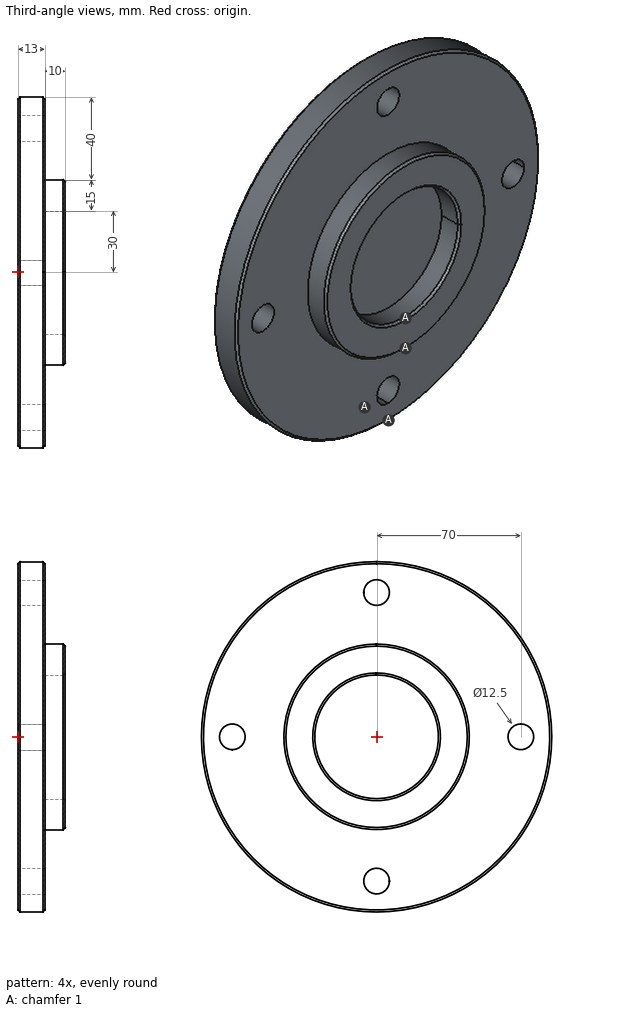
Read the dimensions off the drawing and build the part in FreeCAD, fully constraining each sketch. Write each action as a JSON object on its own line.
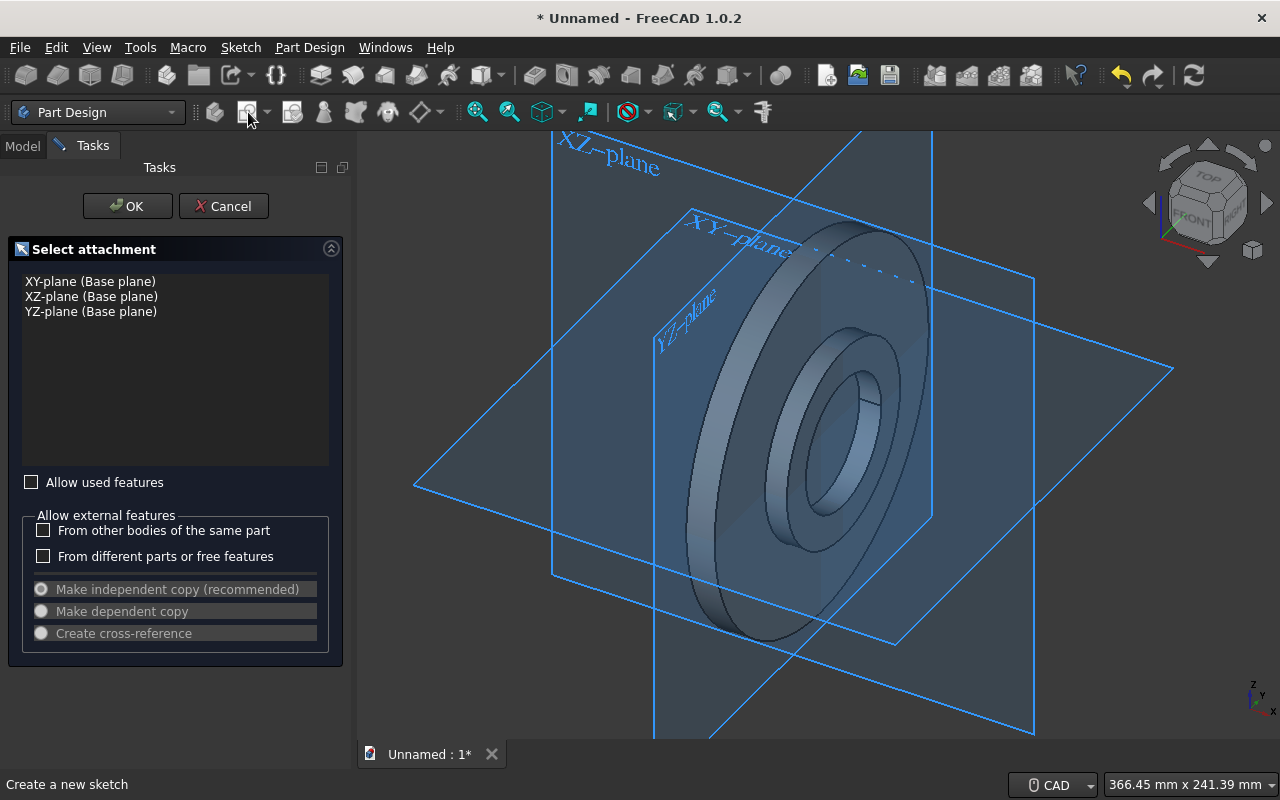
{"action": "left_click", "coordinate": [82, 312]}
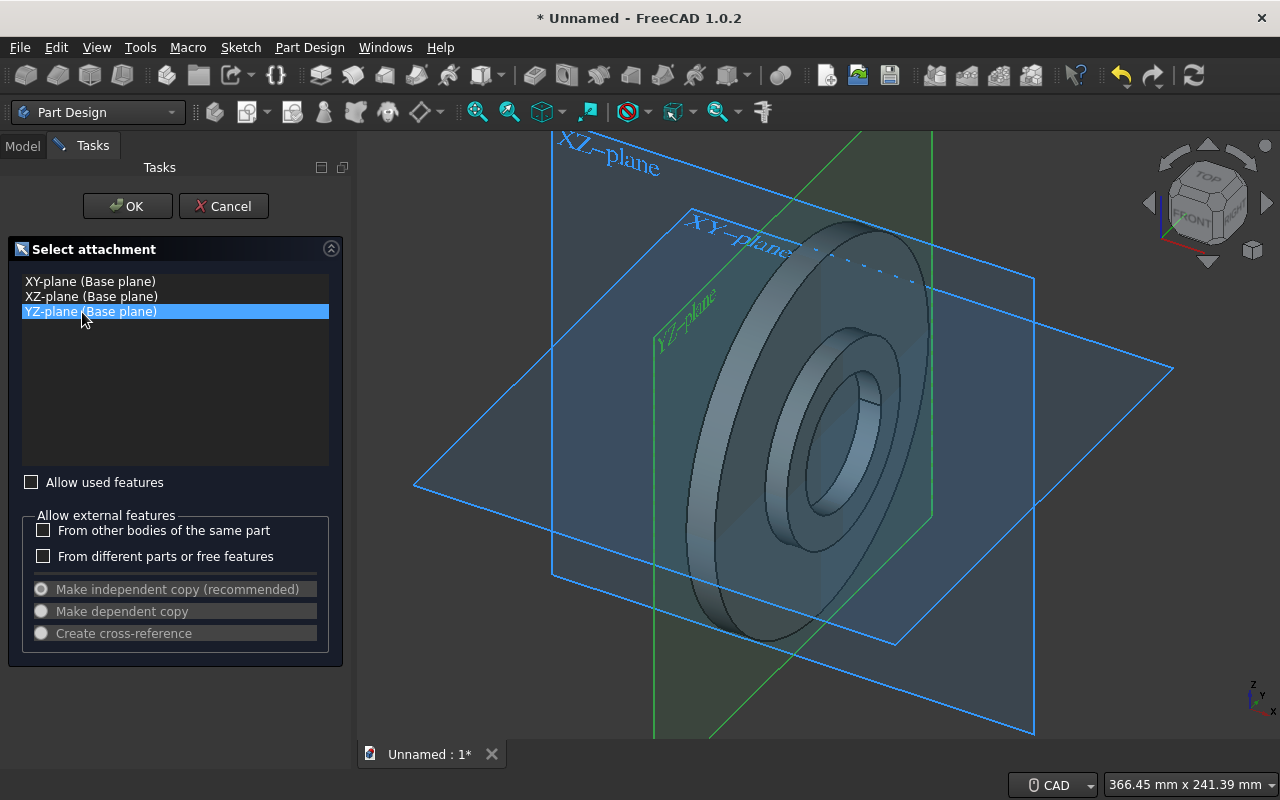
{"action": "left_click", "coordinate": [128, 206]}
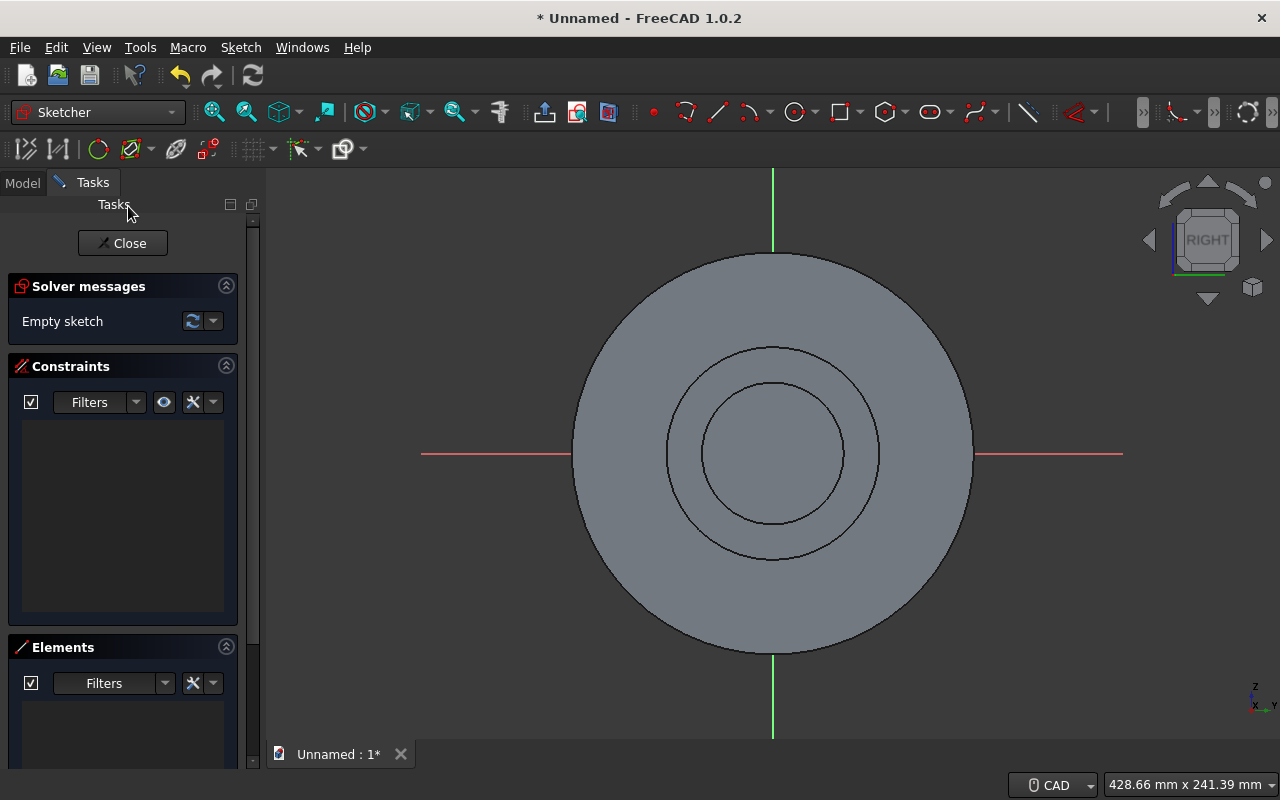
{"action": "key", "text": "q s"}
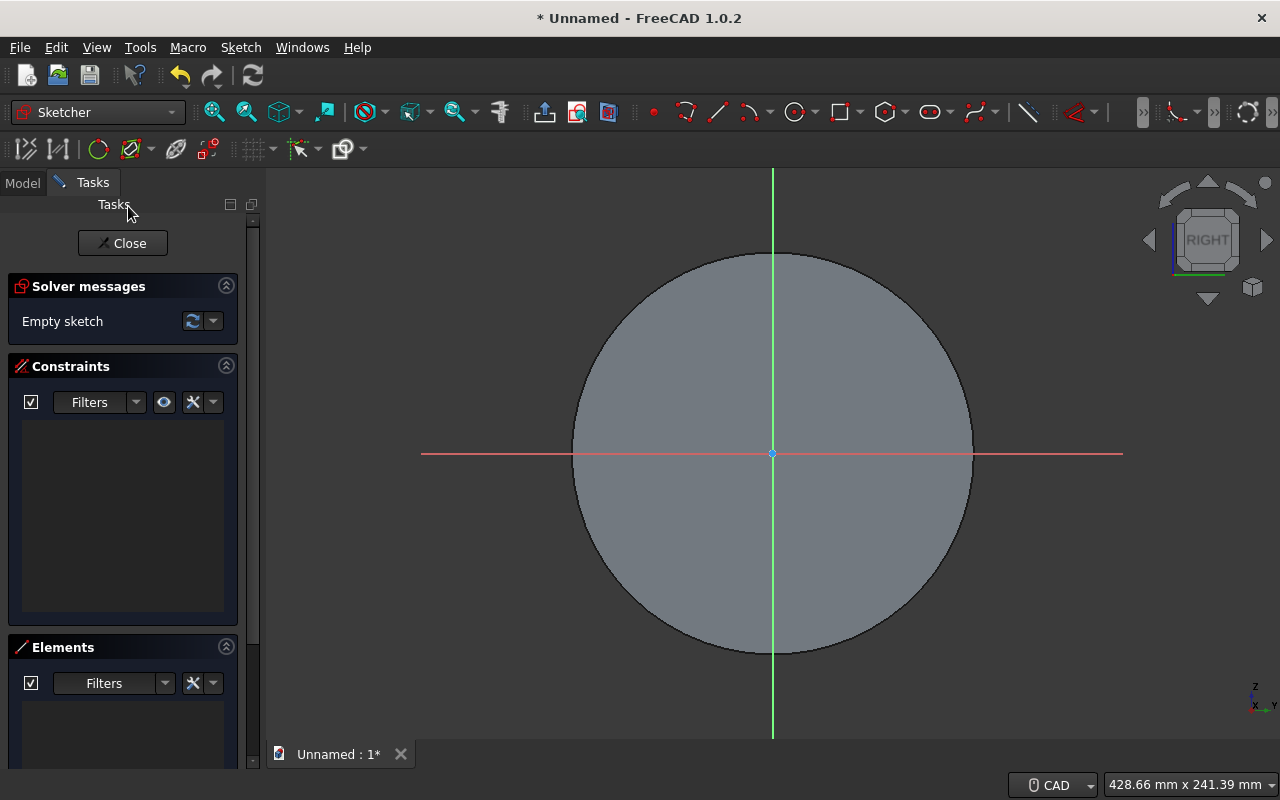
{"action": "scroll", "coordinate": [957, 454], "scroll_direction": "up", "scroll_amount": 13}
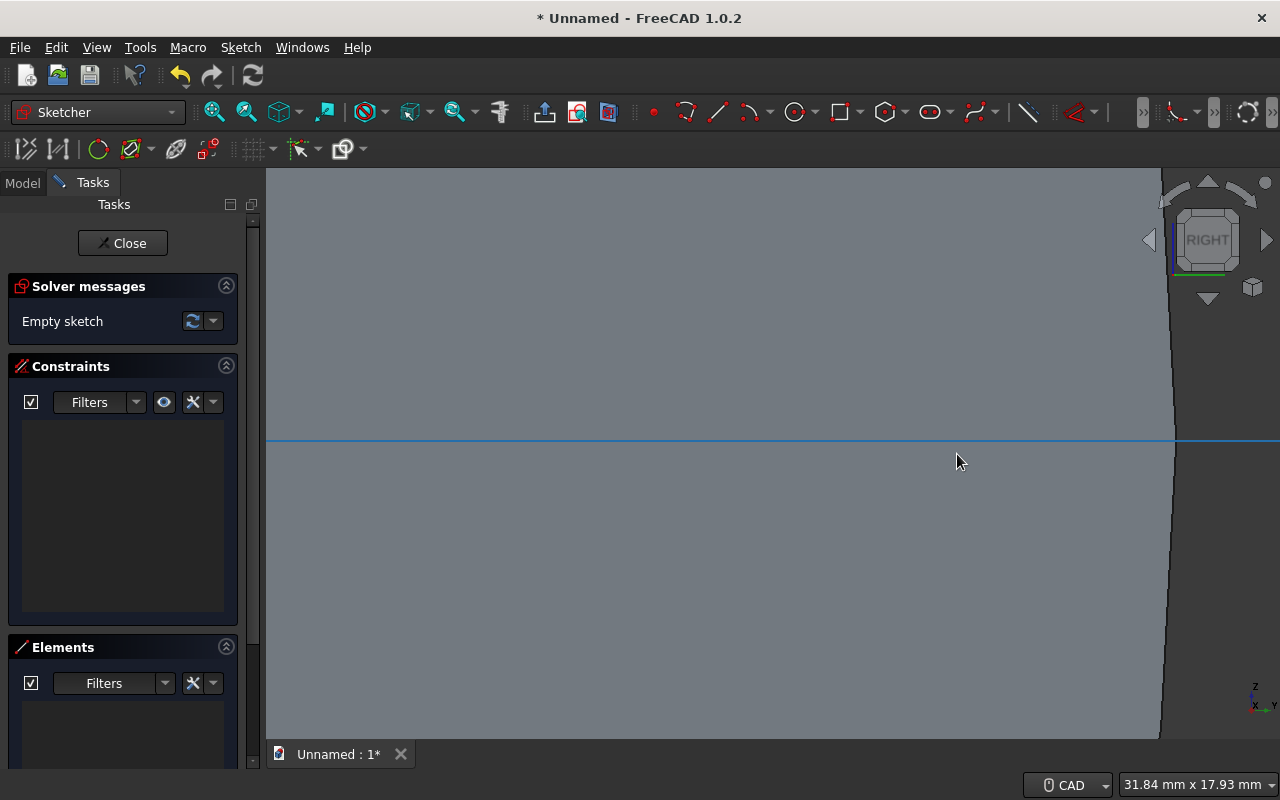
{"action": "left_click", "coordinate": [796, 112]}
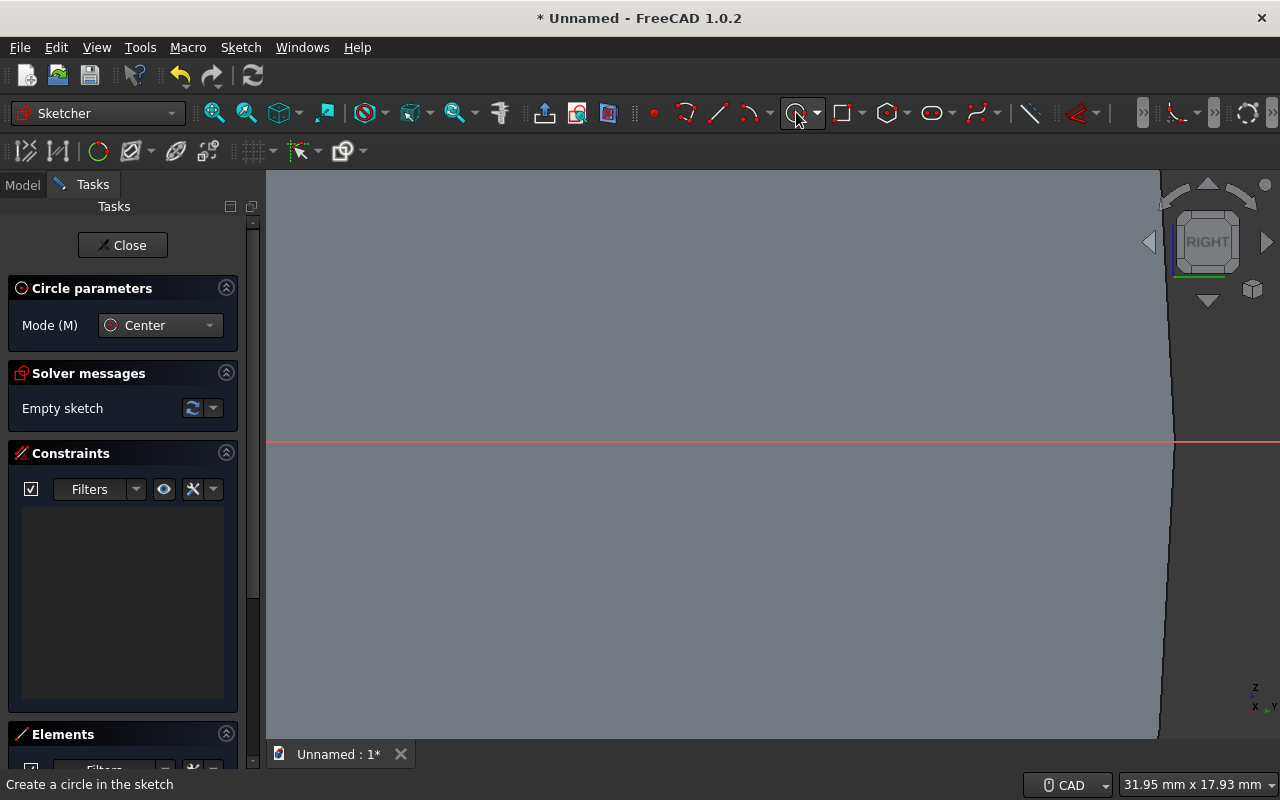
{"action": "left_click", "coordinate": [699, 442]}
{"action": "left_click", "coordinate": [839, 302]}
{"action": "key", "text": "Escape"}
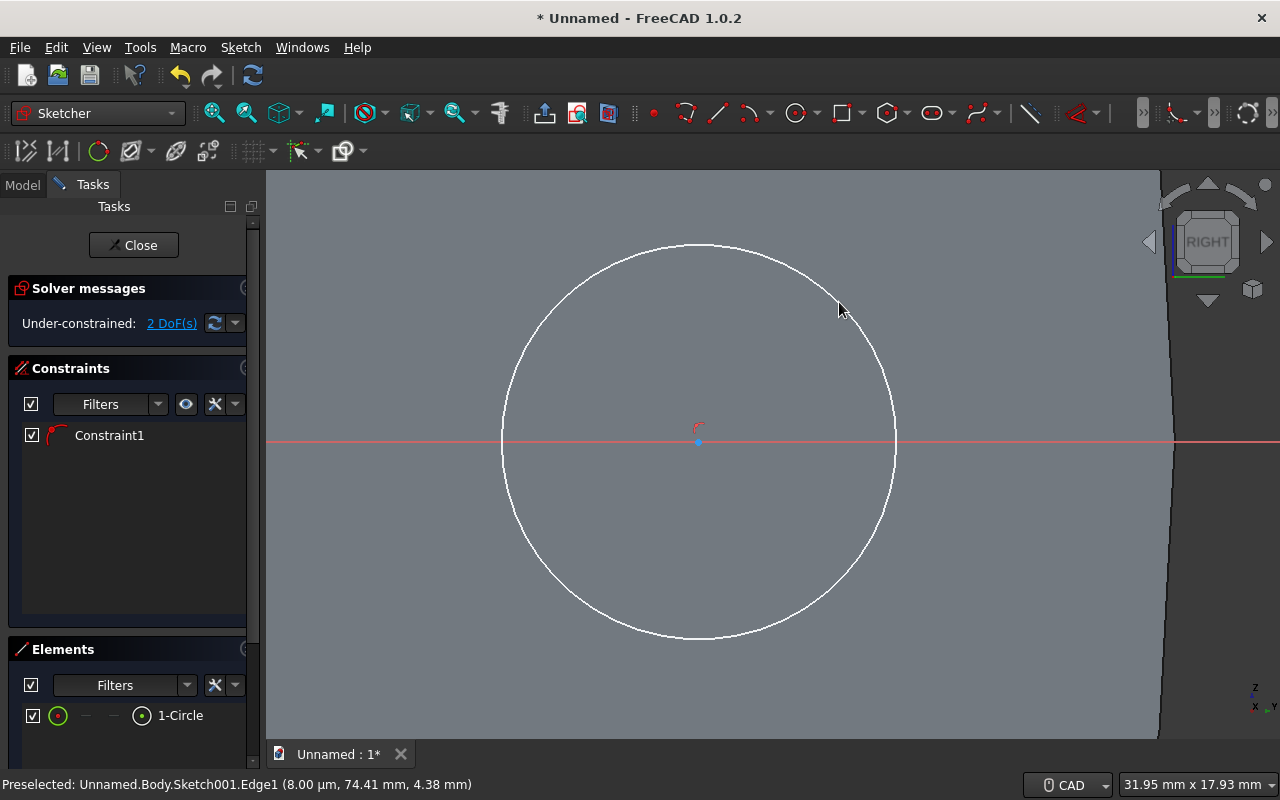
{"action": "key", "text": "d"}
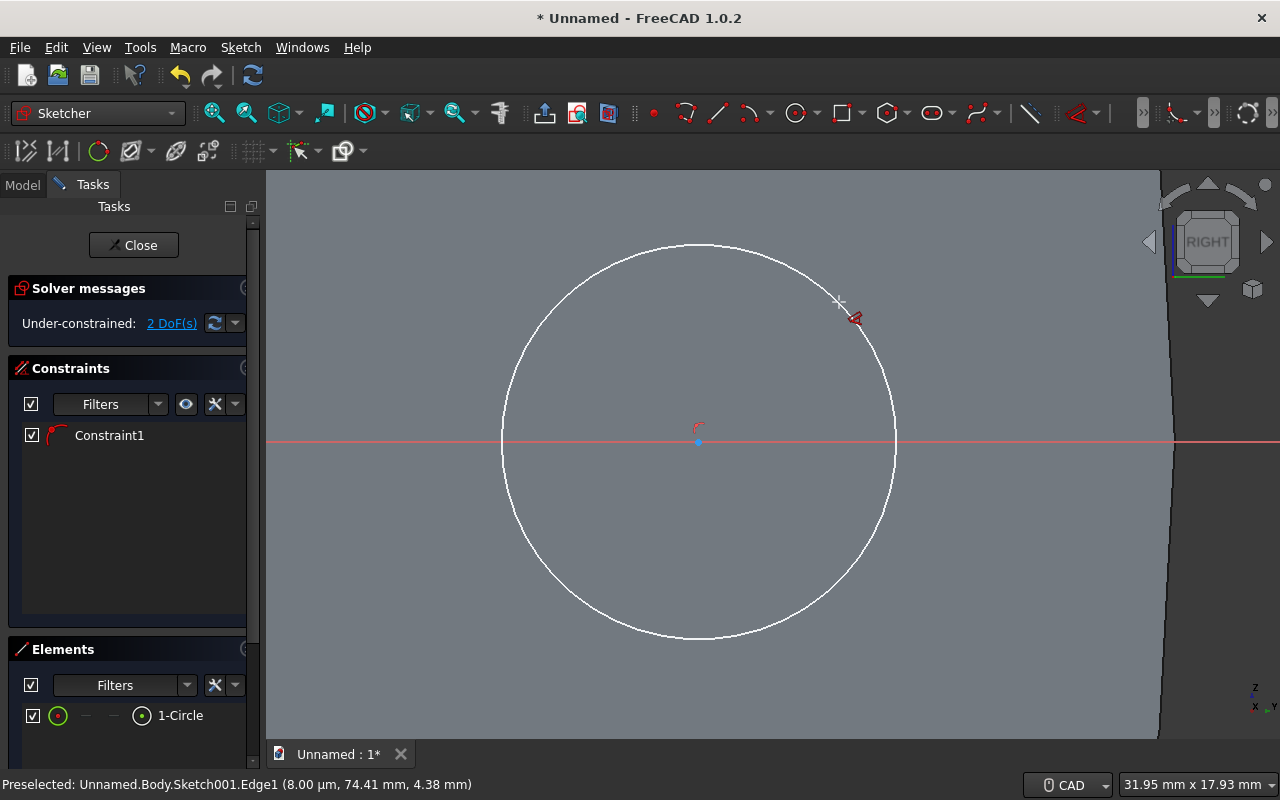
{"action": "left_click", "coordinate": [838, 302]}
{"action": "left_click", "coordinate": [861, 279]}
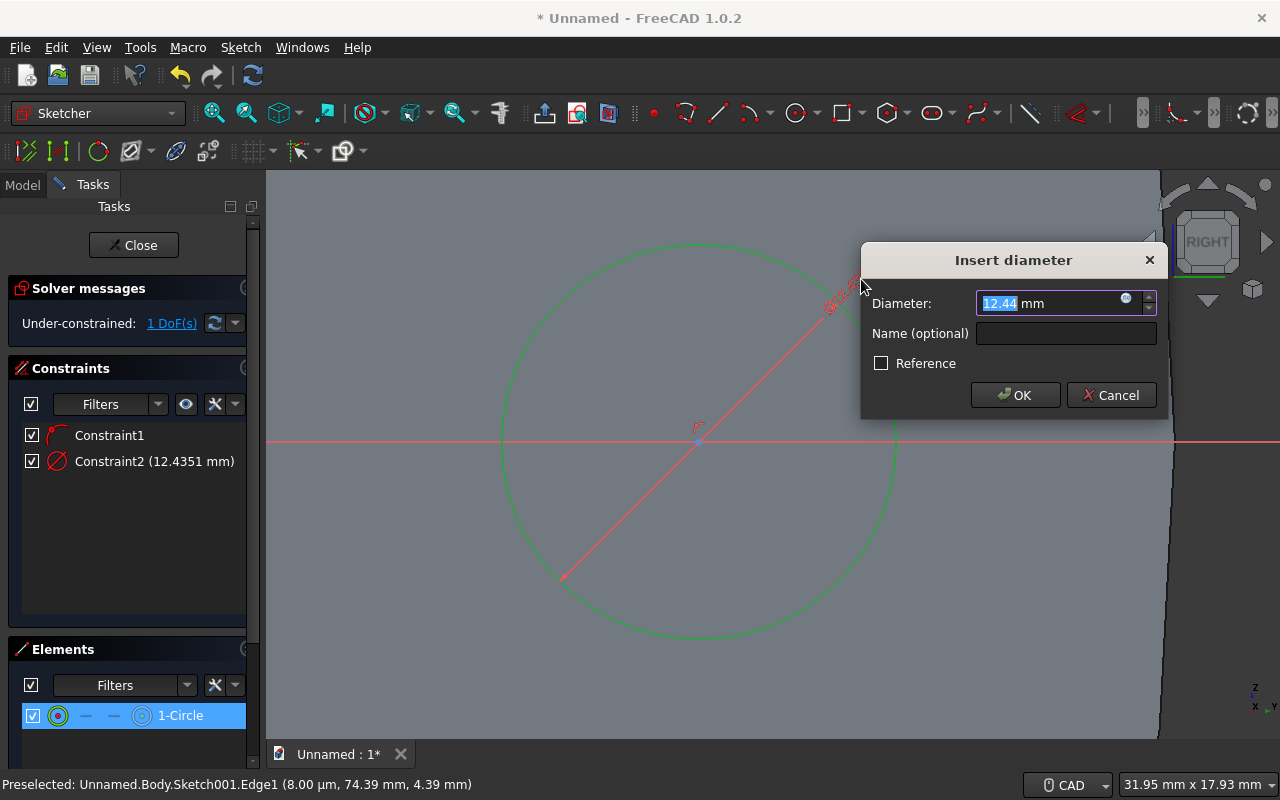
{"action": "type", "text": "12.5"}
{"action": "key", "text": "Return"}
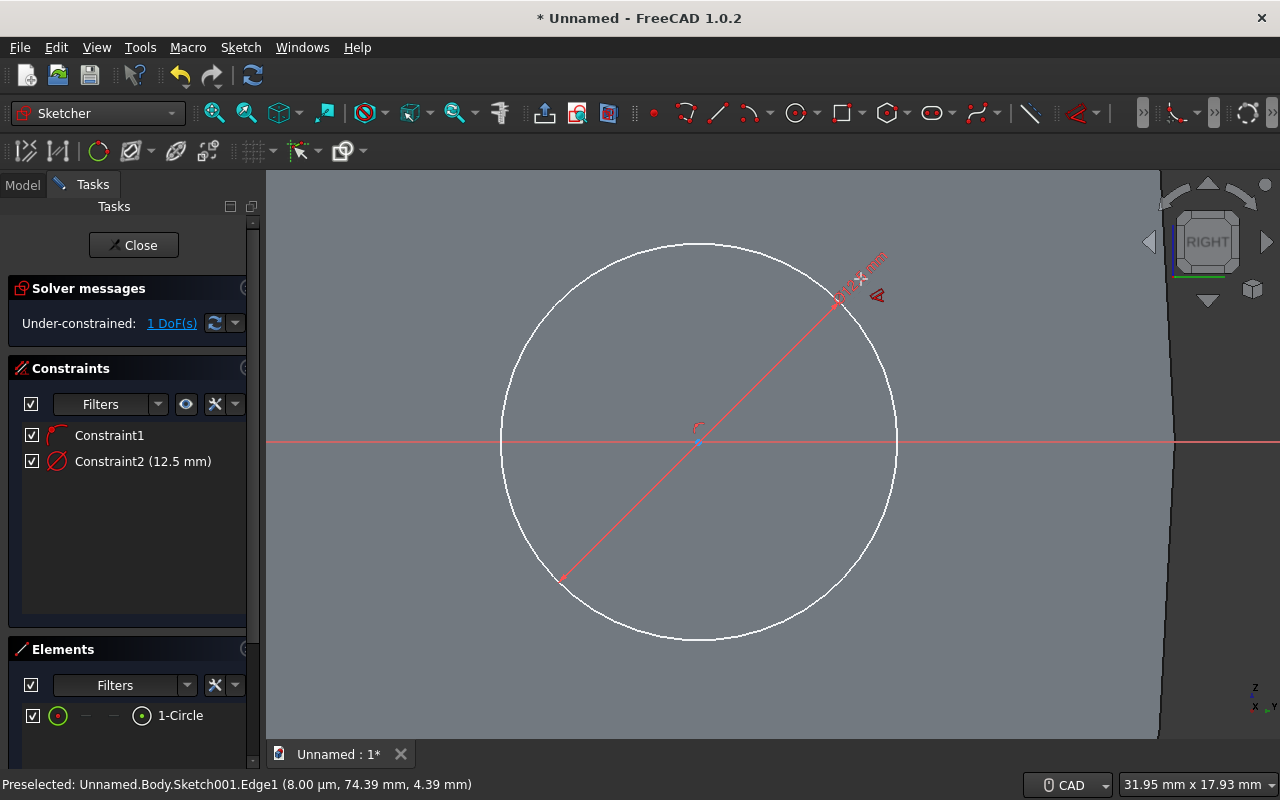
{"action": "left_click", "coordinate": [699, 442]}
{"action": "left_click", "coordinate": [403, 476]}